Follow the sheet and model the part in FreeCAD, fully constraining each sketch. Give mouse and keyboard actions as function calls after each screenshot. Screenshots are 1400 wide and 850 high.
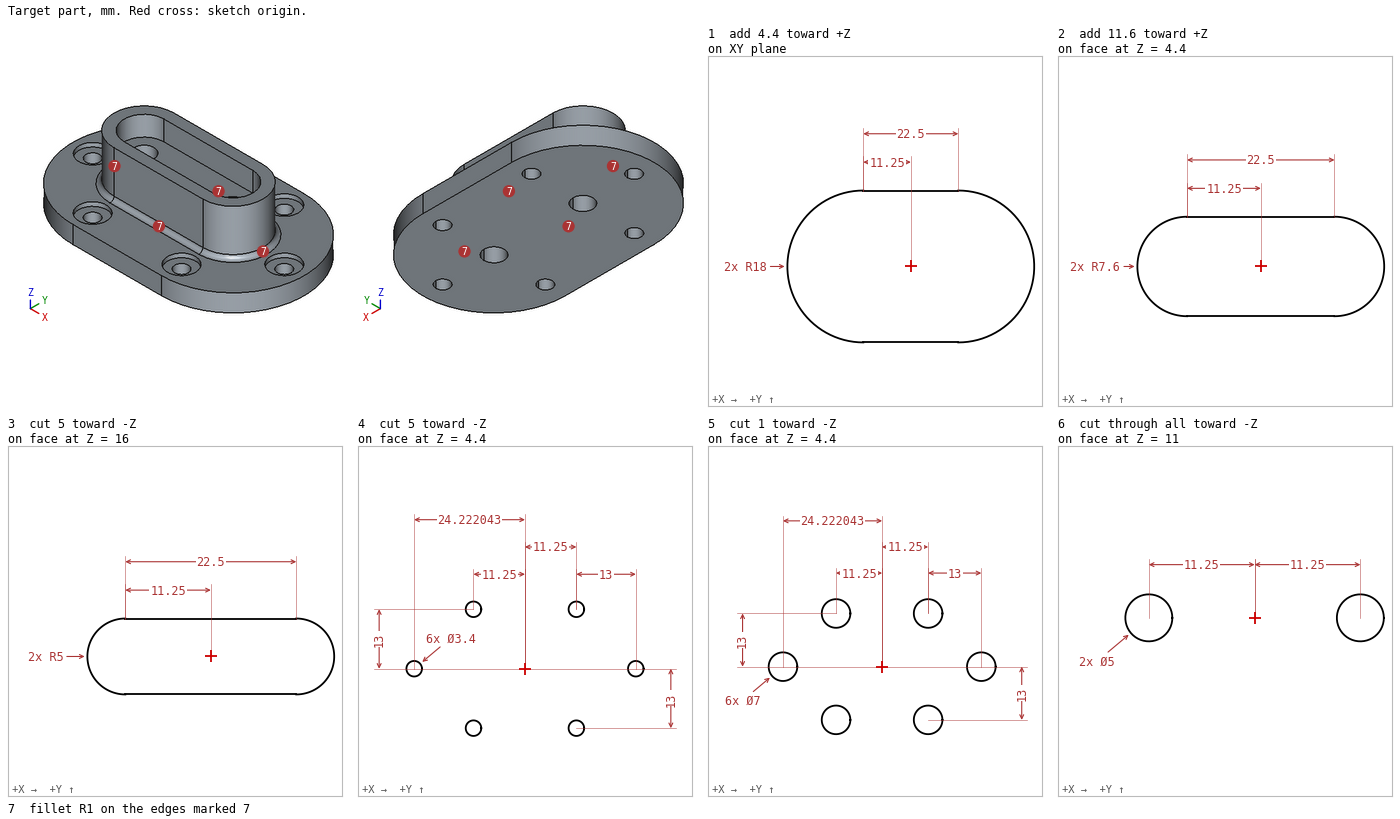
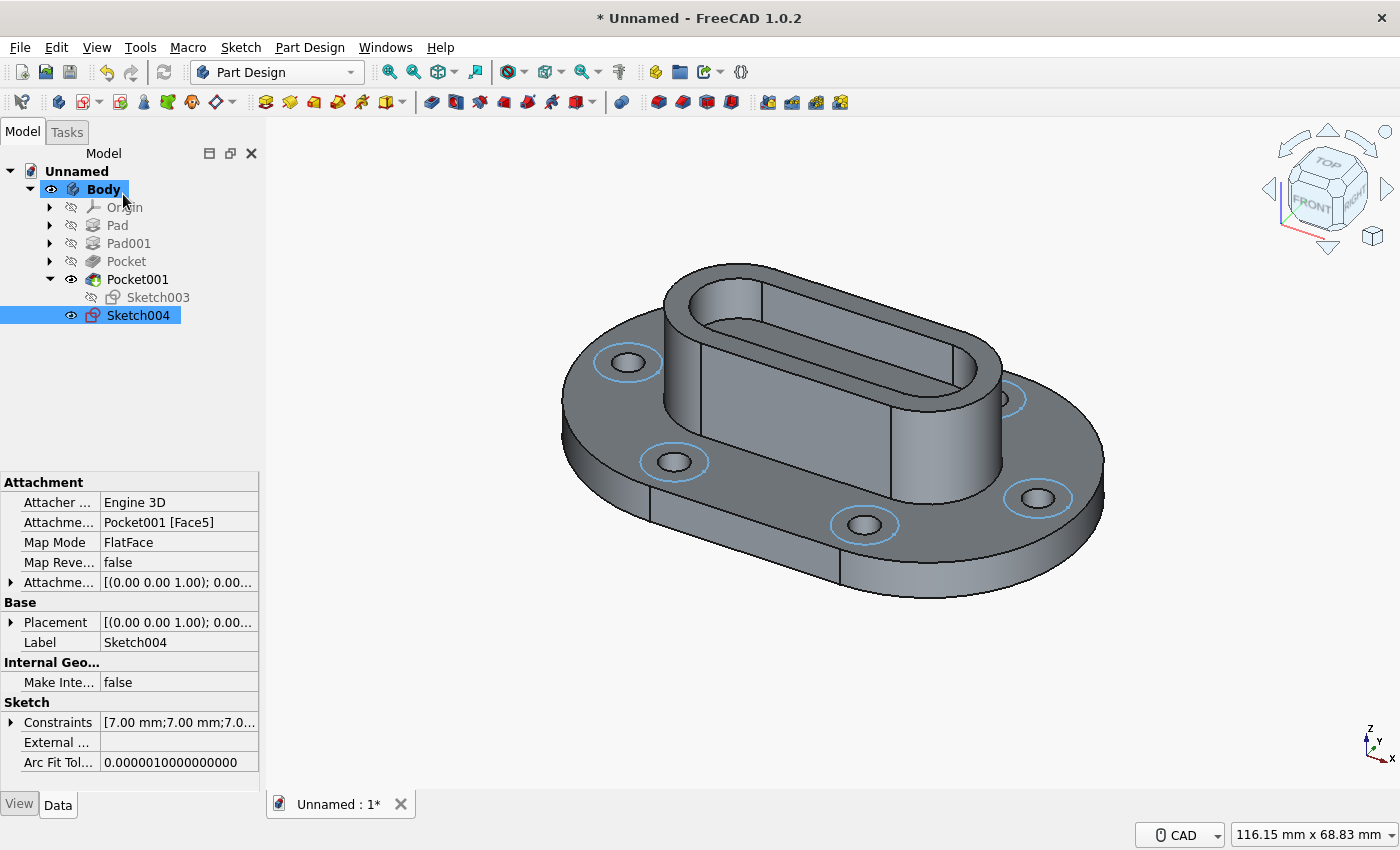
click(432, 102)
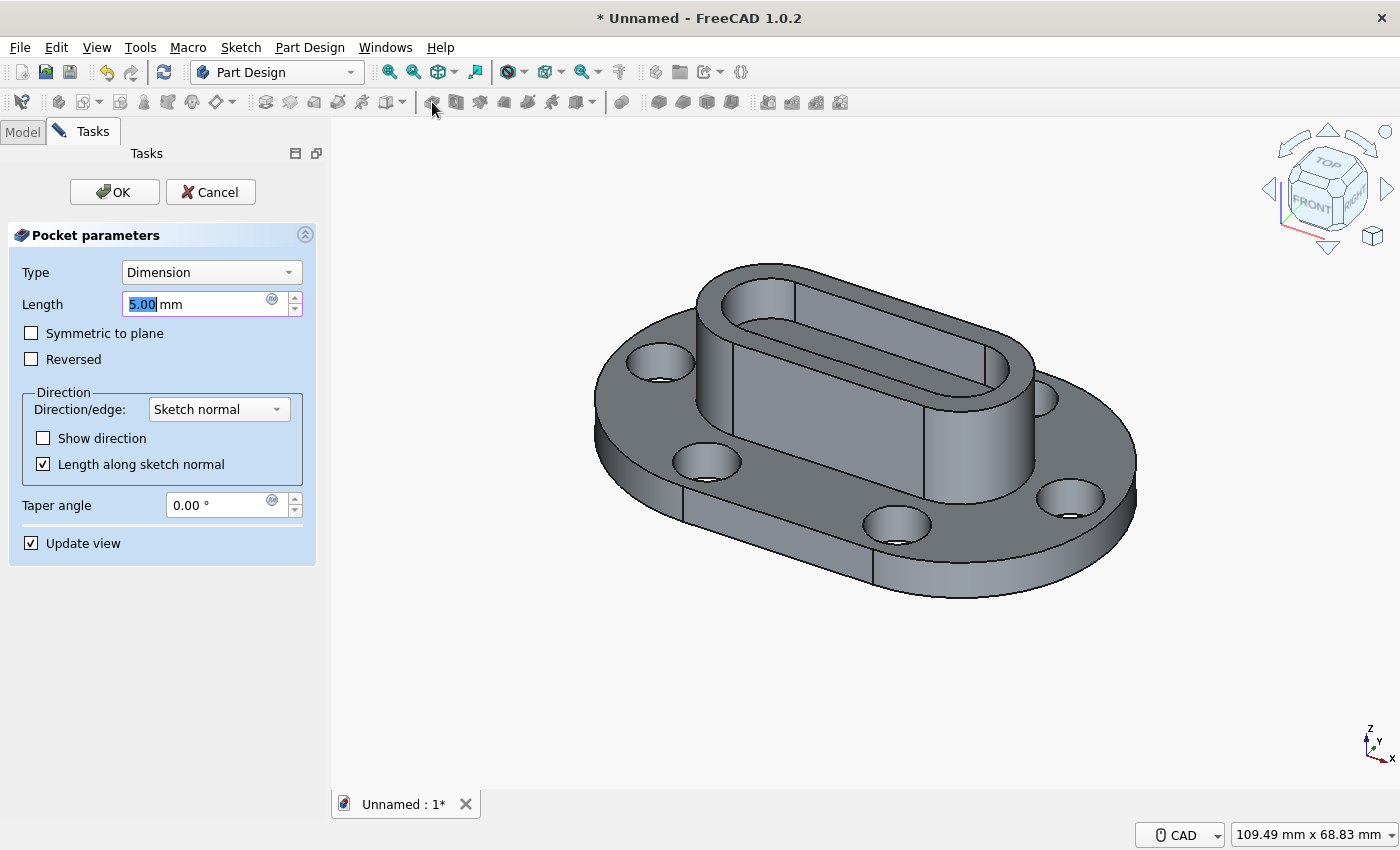
text(1)
key(Tab)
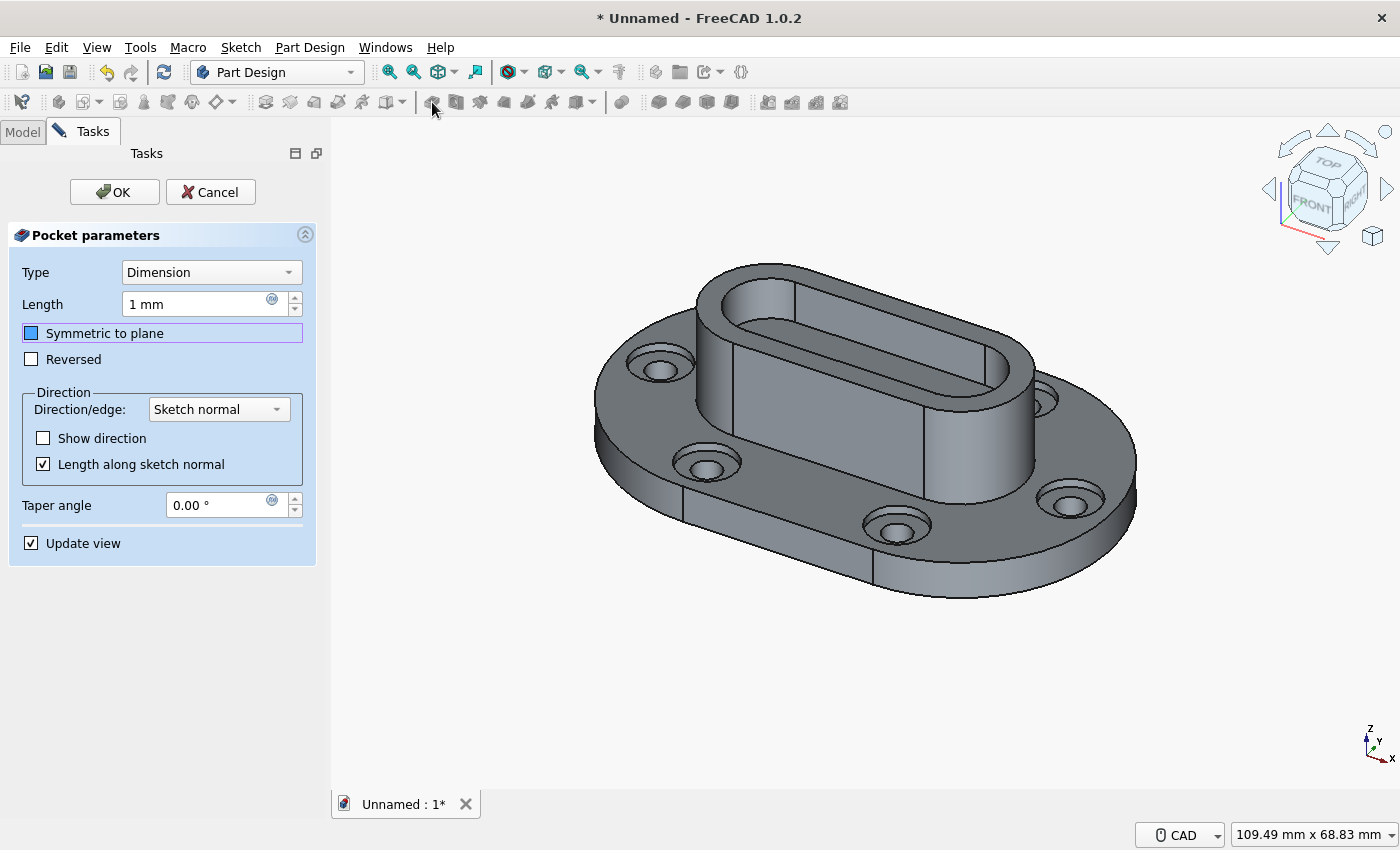
click(115, 192)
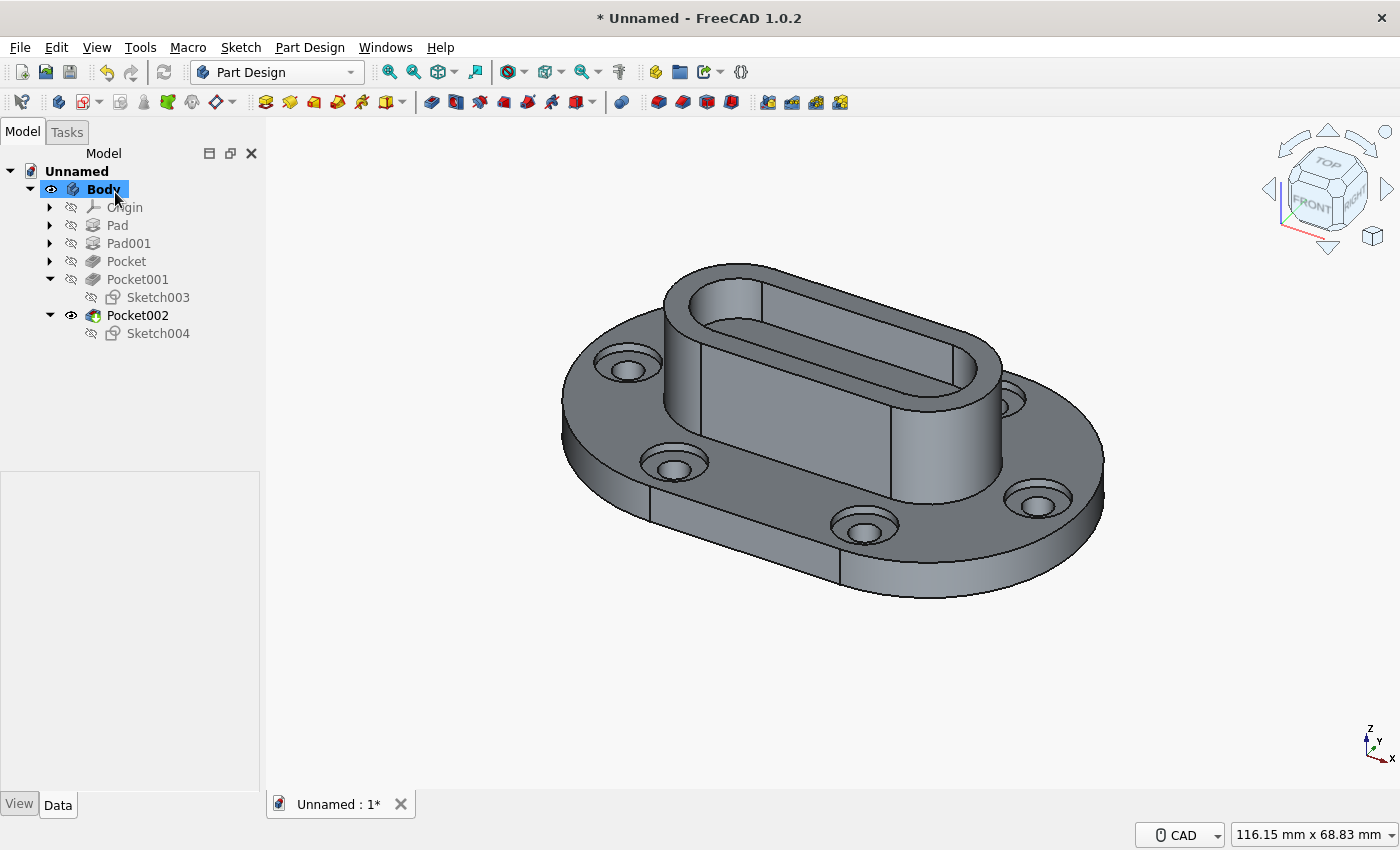
key(0)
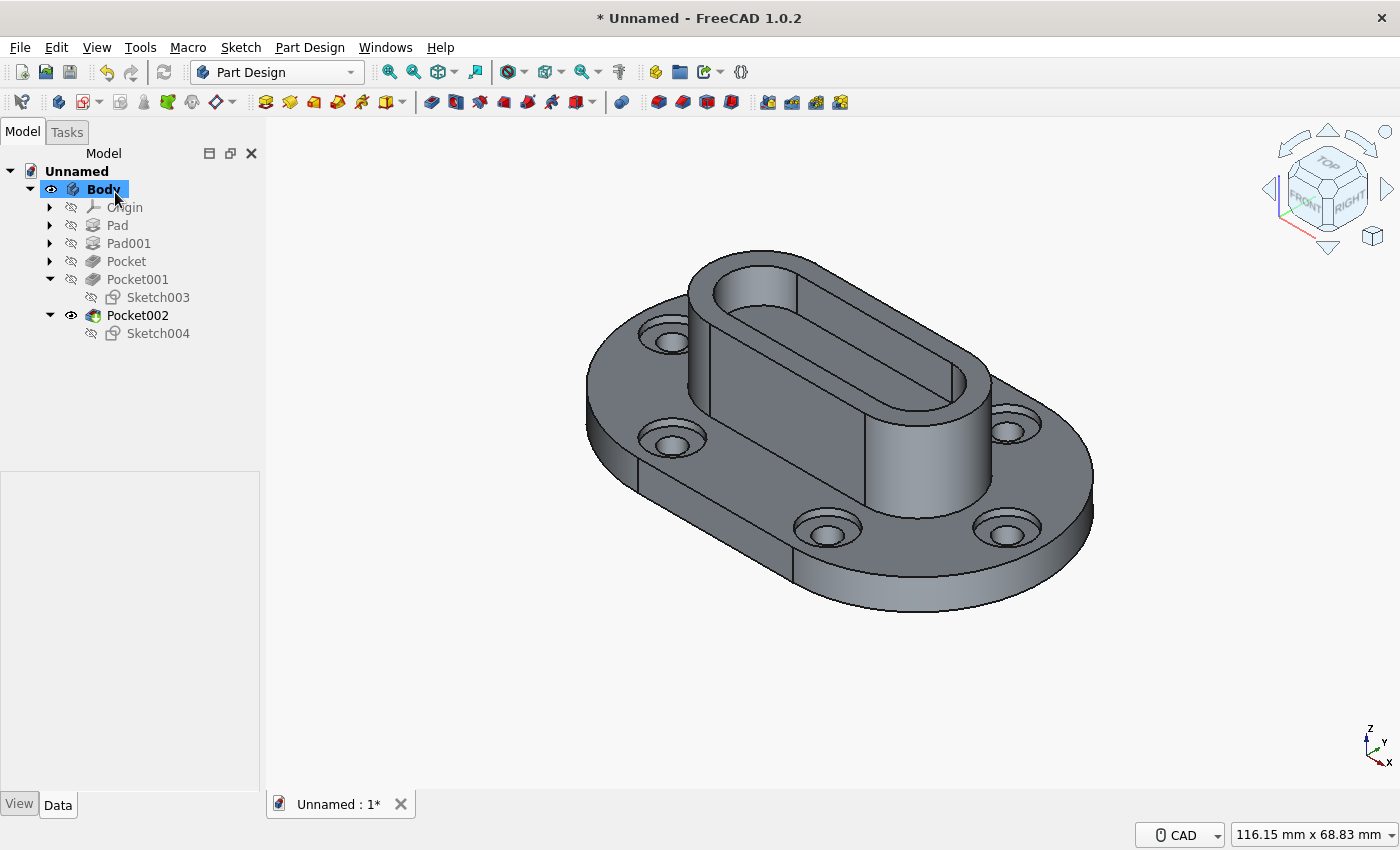
key(2)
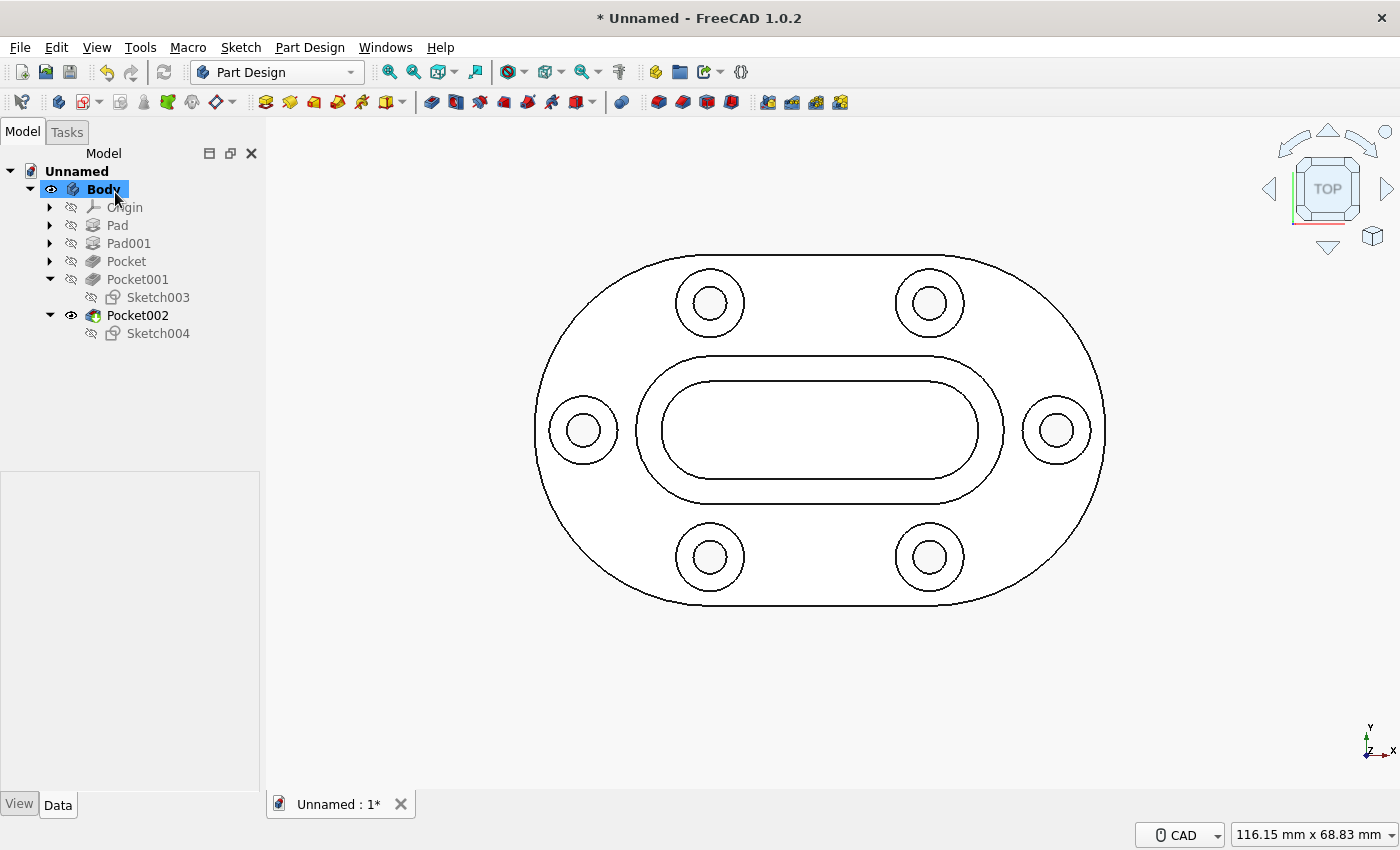
click(911, 429)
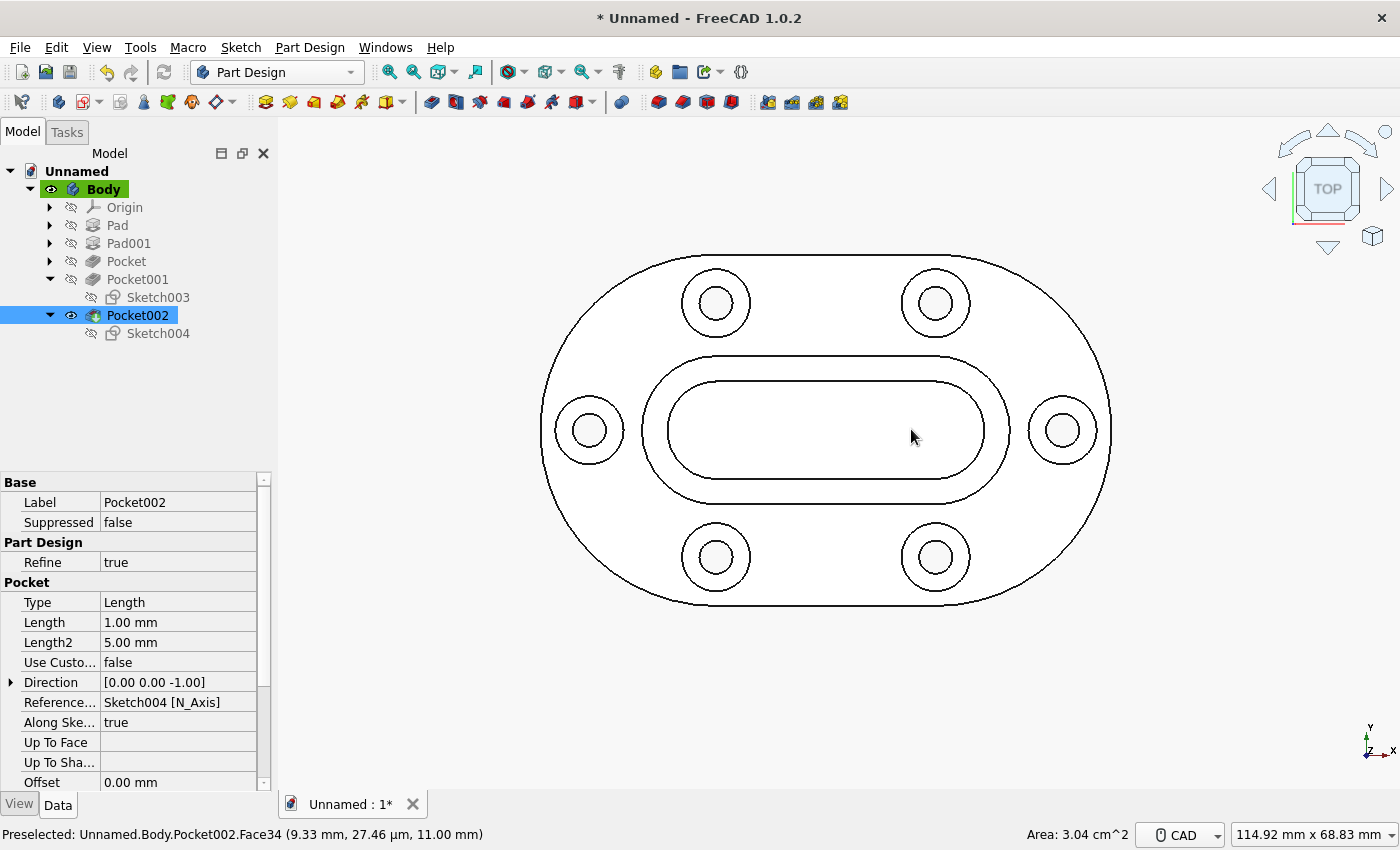
click(84, 102)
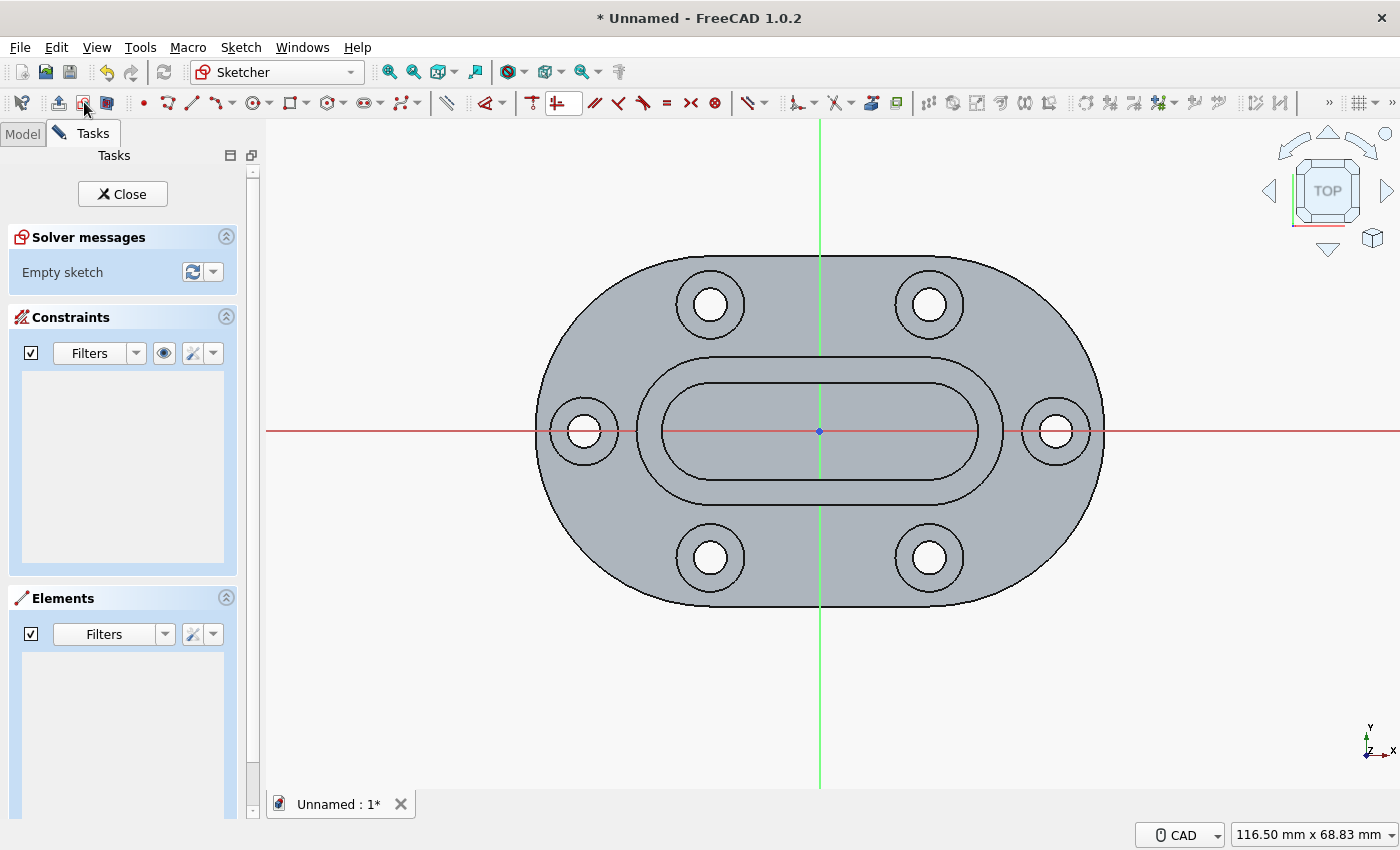
scroll(852, 418, up, 5)